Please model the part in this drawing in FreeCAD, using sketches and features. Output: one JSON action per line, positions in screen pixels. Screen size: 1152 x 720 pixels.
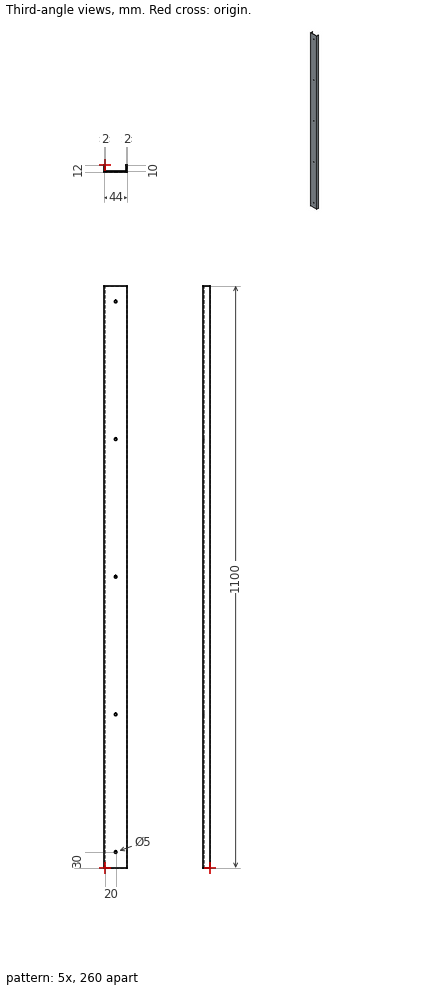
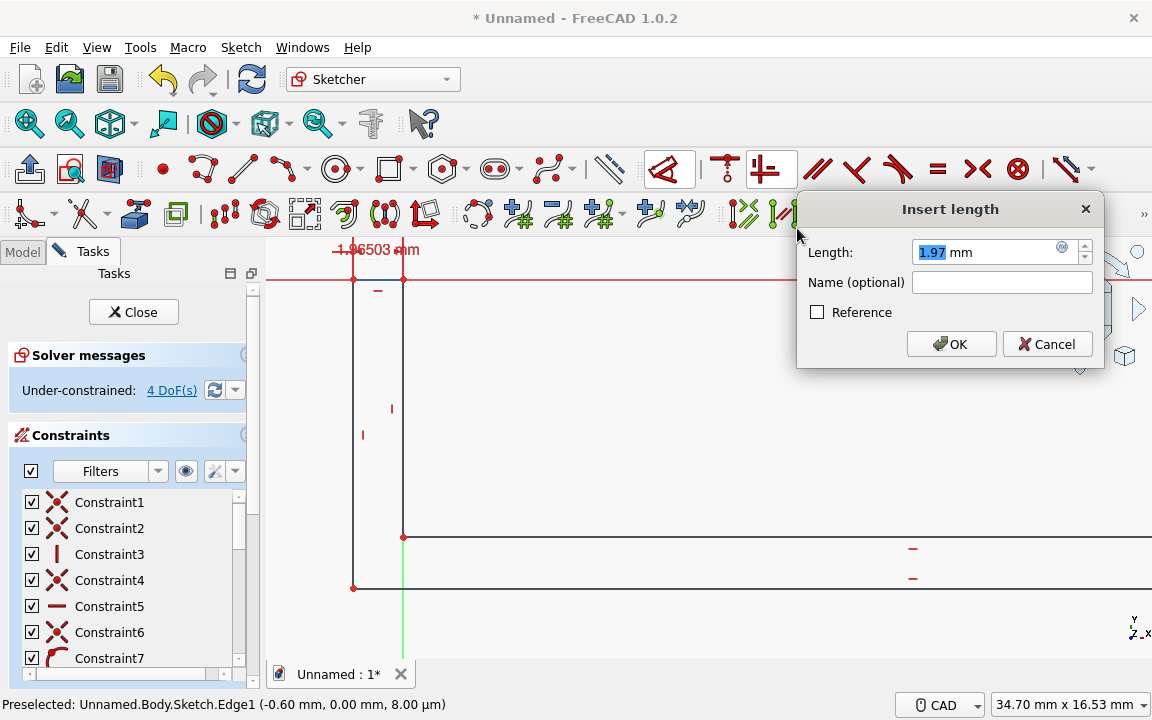
{"action": "type", "text": "2"}
{"action": "key", "text": "Return"}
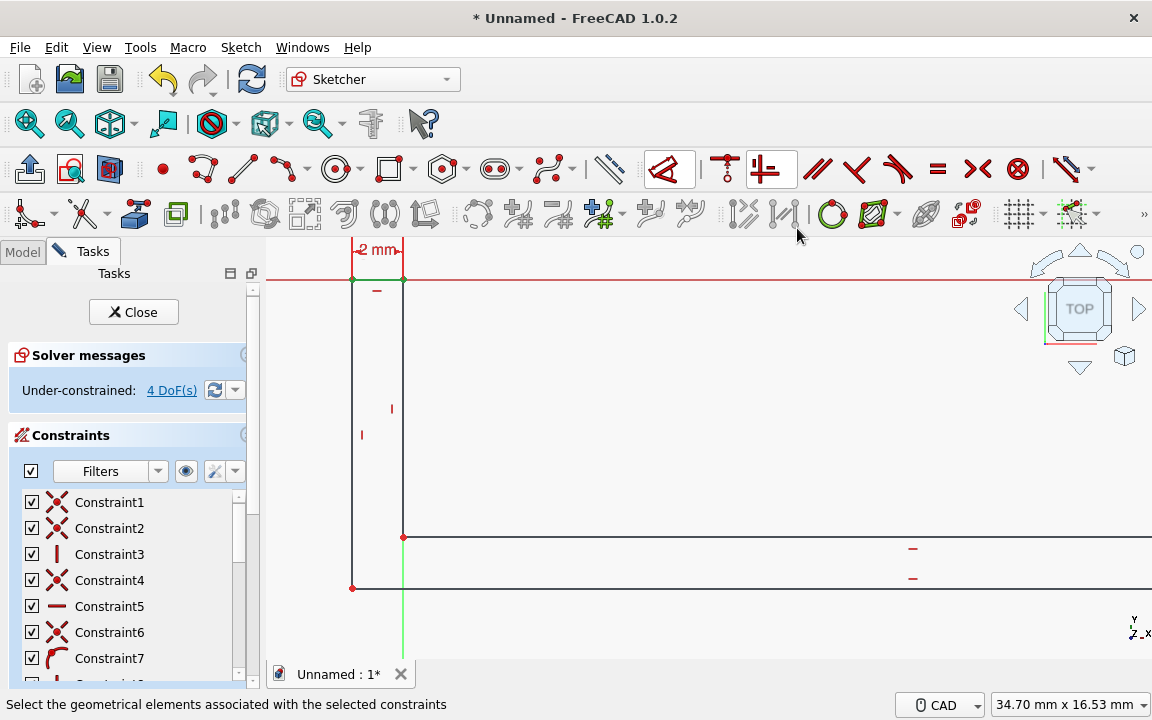
{"action": "scroll", "coordinate": [418, 460], "scroll_direction": "down", "scroll_amount": 4}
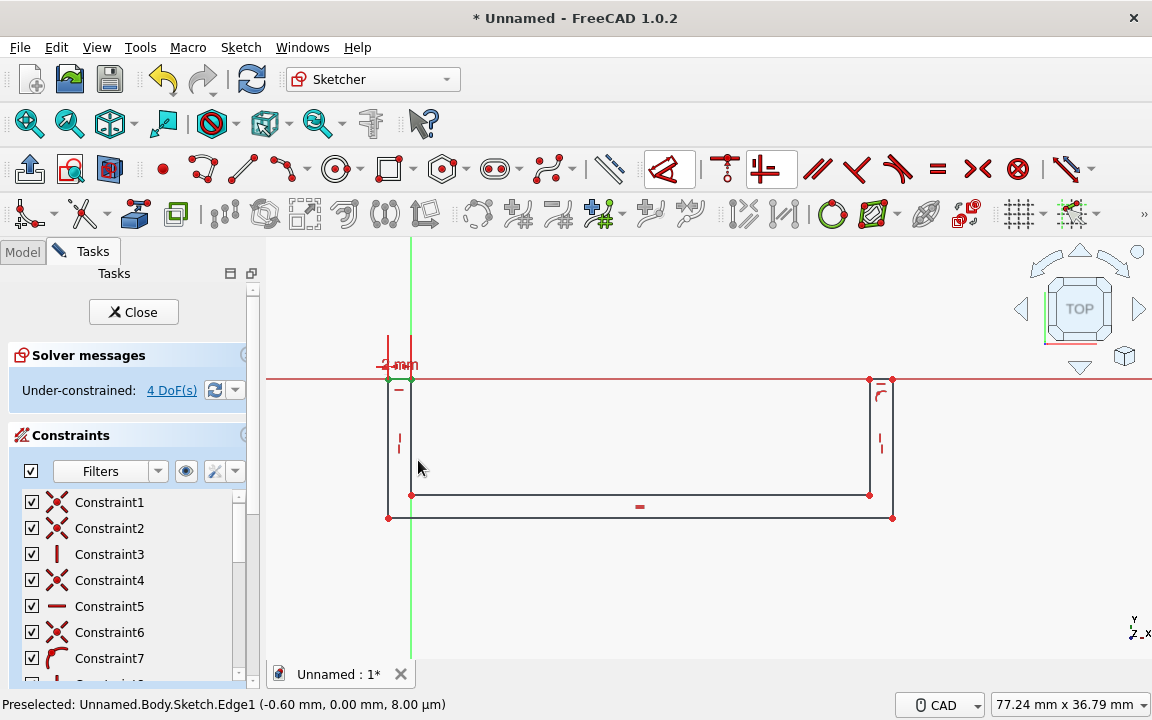
{"action": "scroll", "coordinate": [886, 379], "scroll_direction": "up", "scroll_amount": 4}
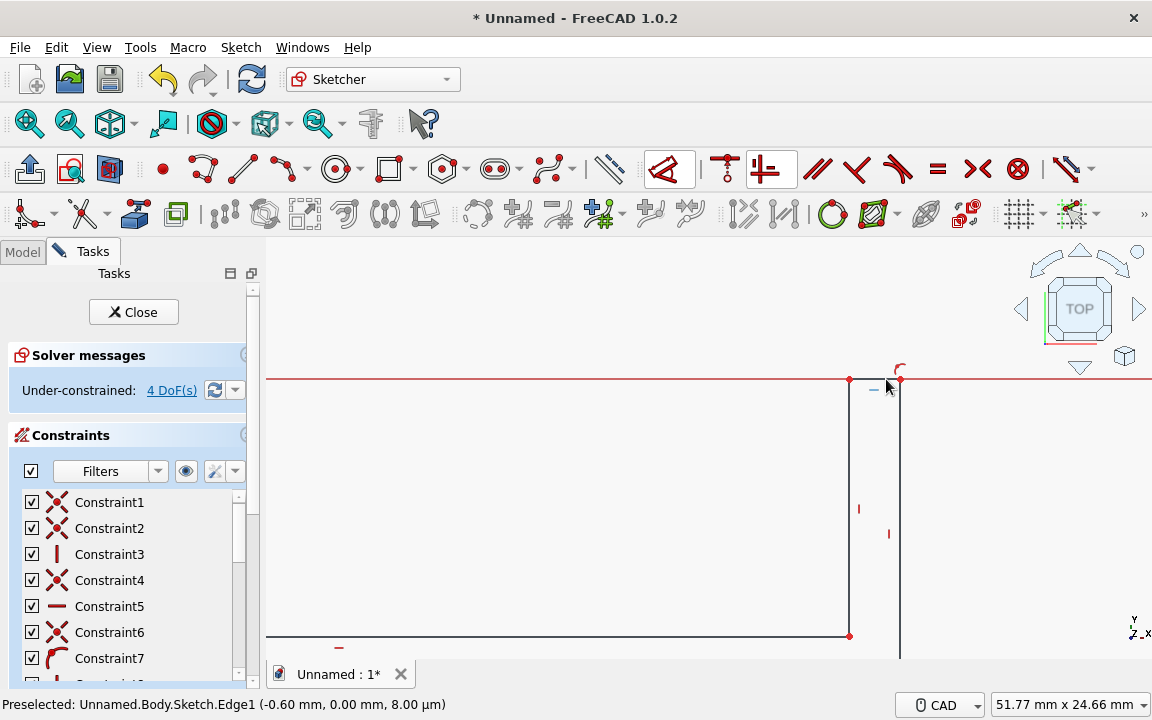
{"action": "left_click", "coordinate": [885, 379]}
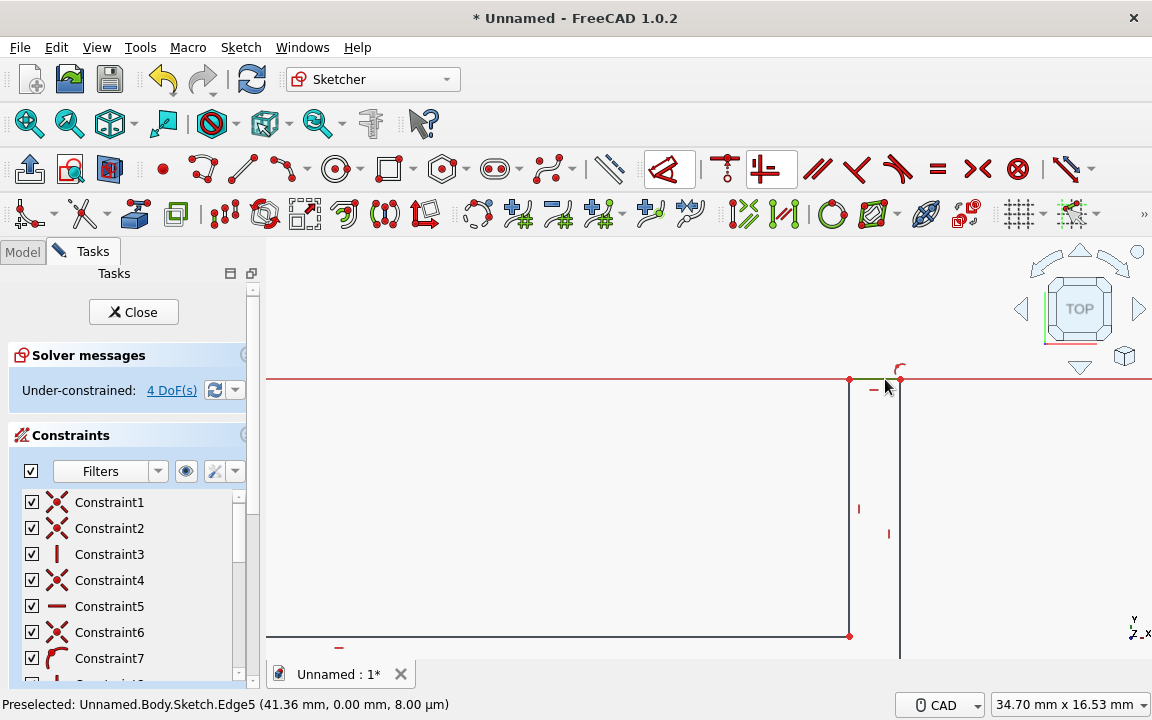
{"action": "key", "text": "l"}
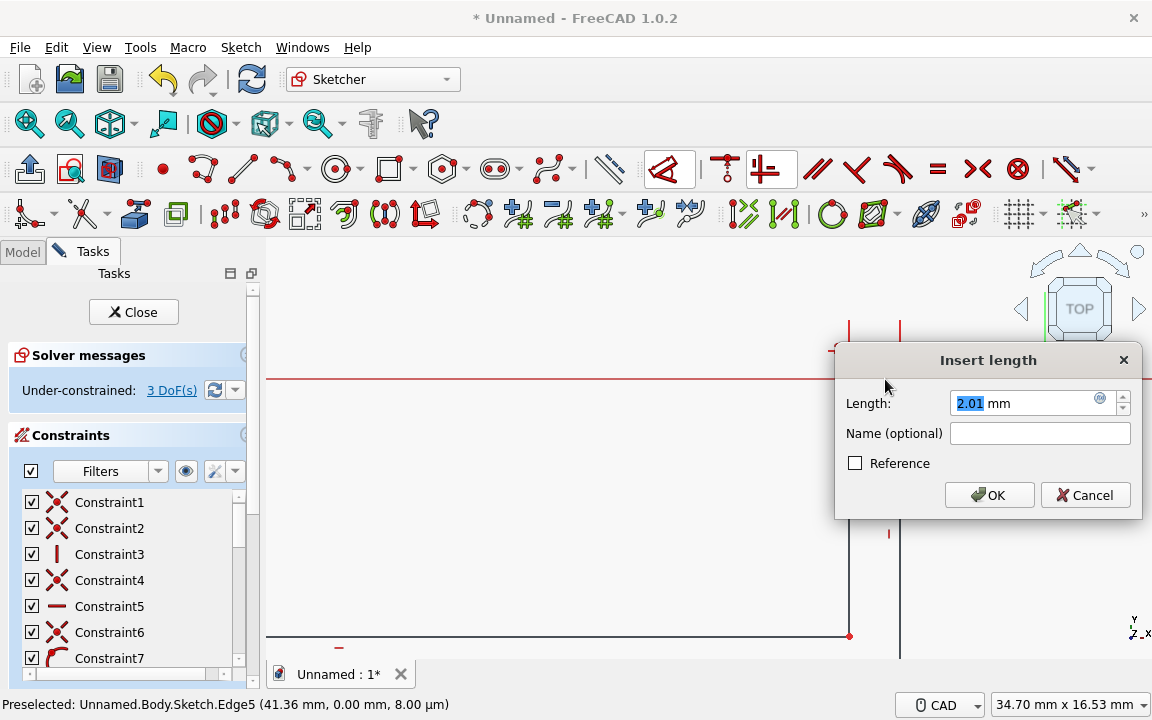
{"action": "type", "text": "2"}
{"action": "key", "text": "Return"}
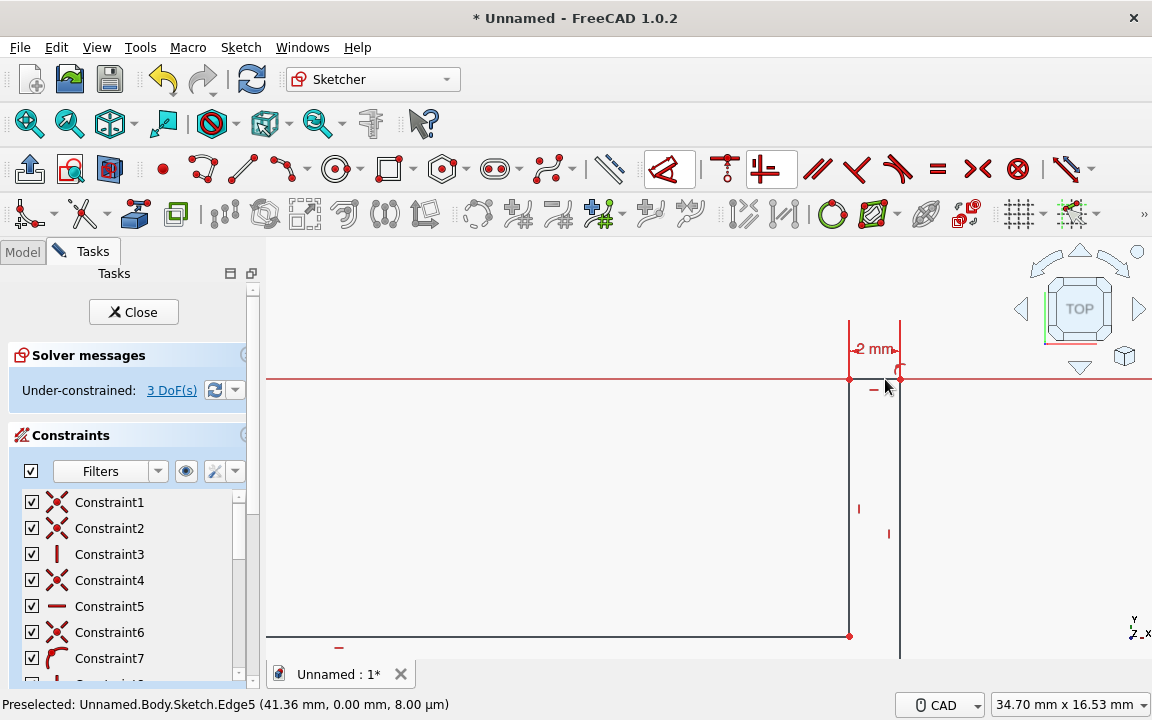
{"action": "scroll", "coordinate": [886, 379], "scroll_direction": "down", "scroll_amount": 4}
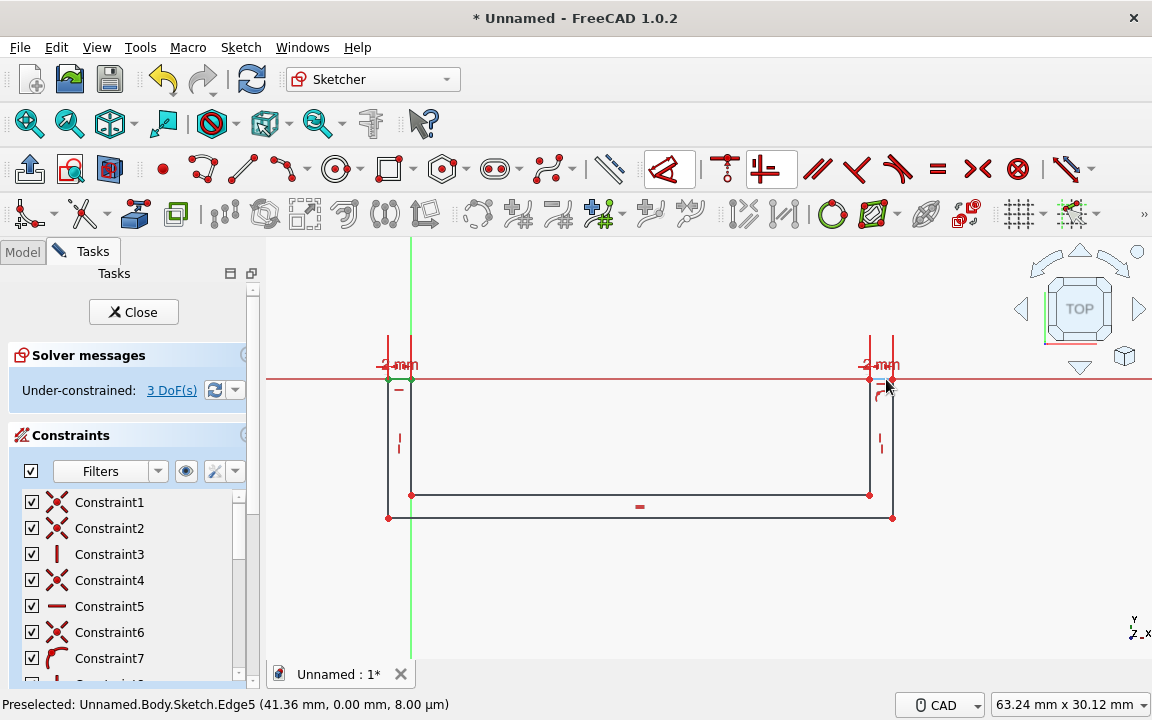
{"action": "left_click", "coordinate": [388, 421]}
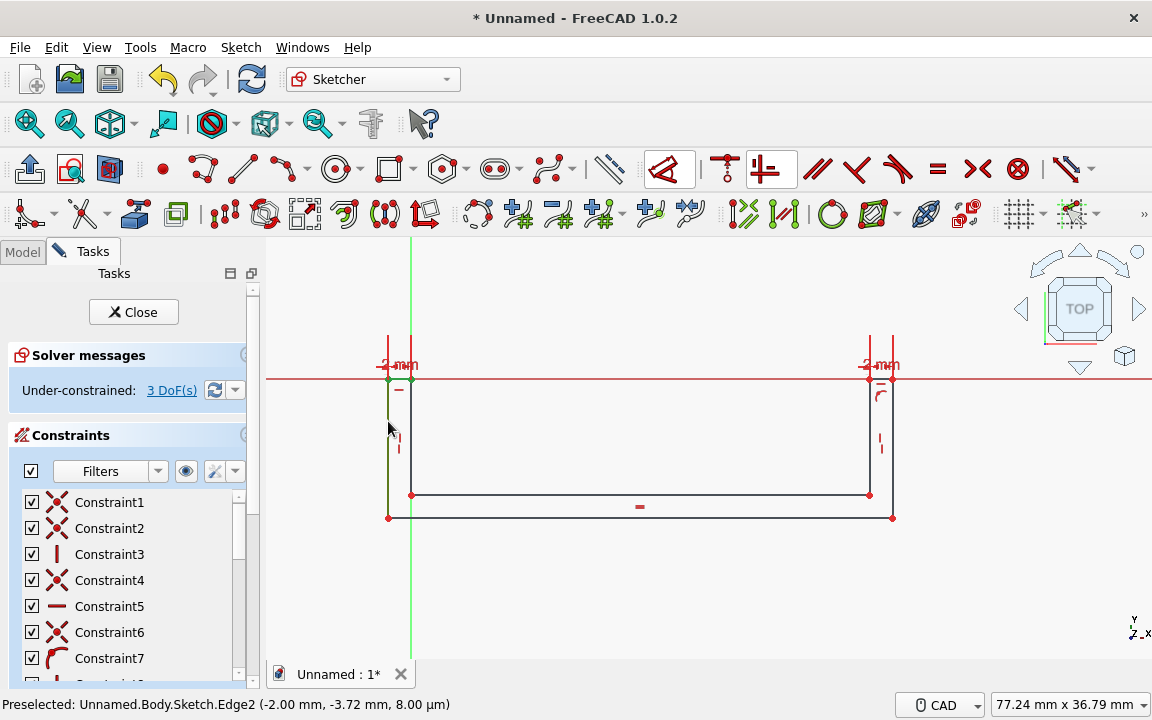
{"action": "left_click", "coordinate": [690, 170]}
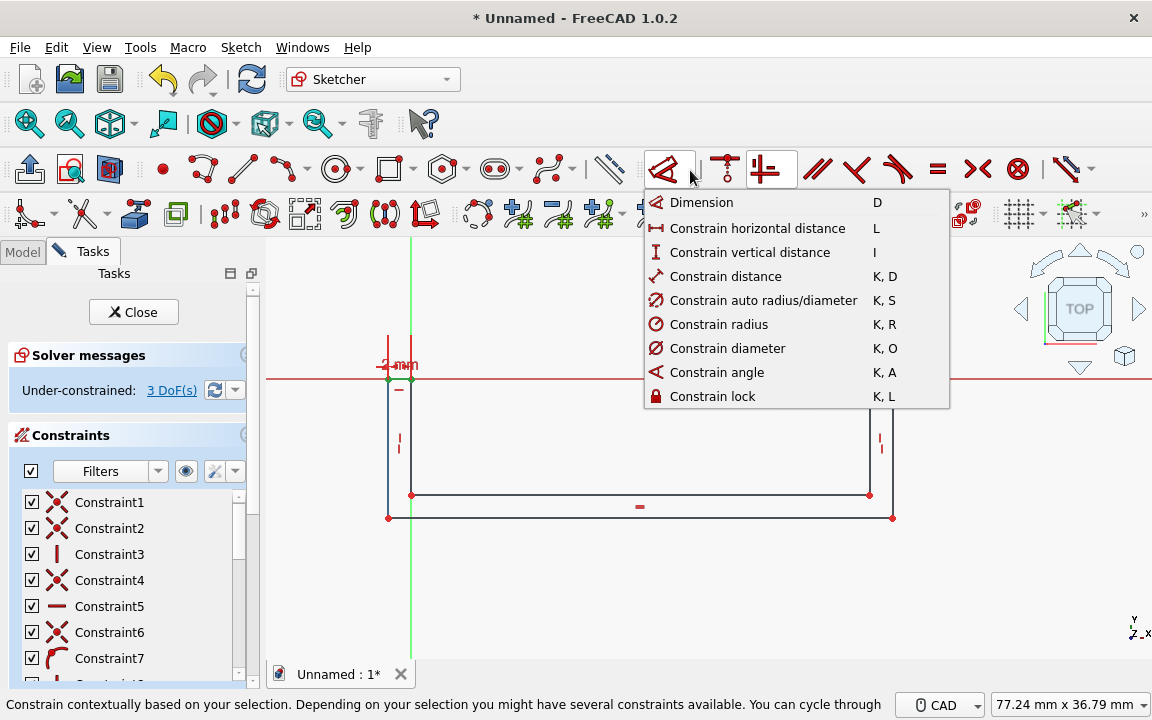
{"action": "left_click", "coordinate": [797, 252]}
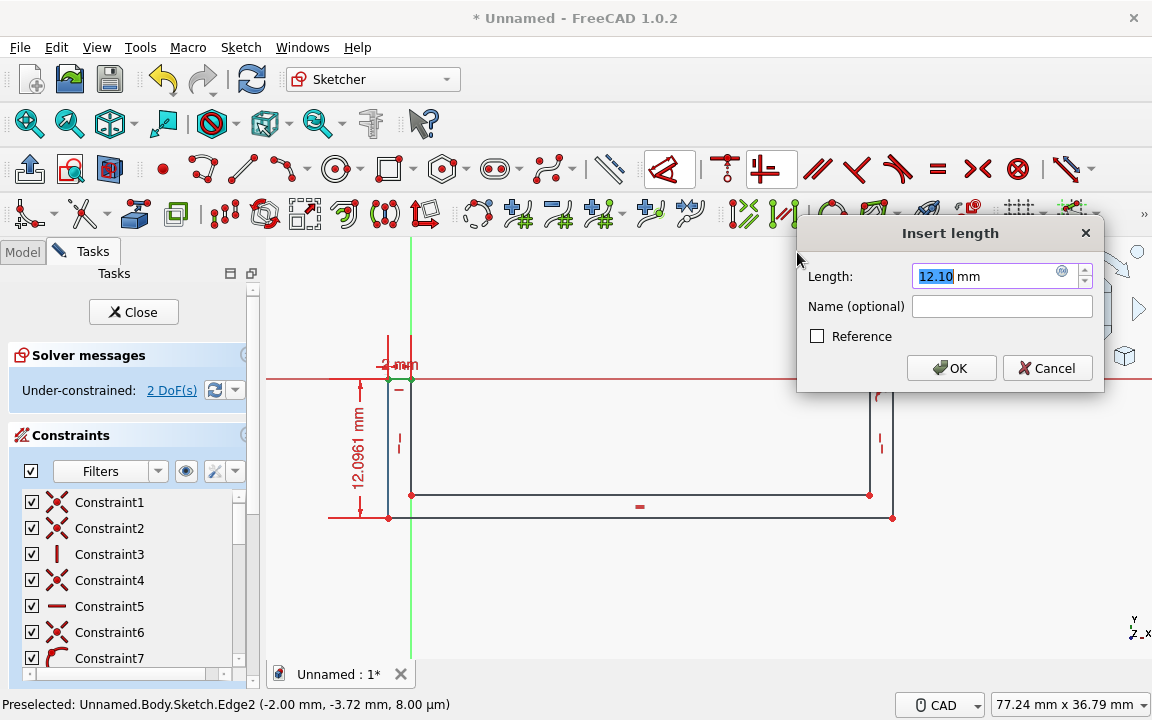
{"action": "type", "text": "12"}
{"action": "key", "text": "Return"}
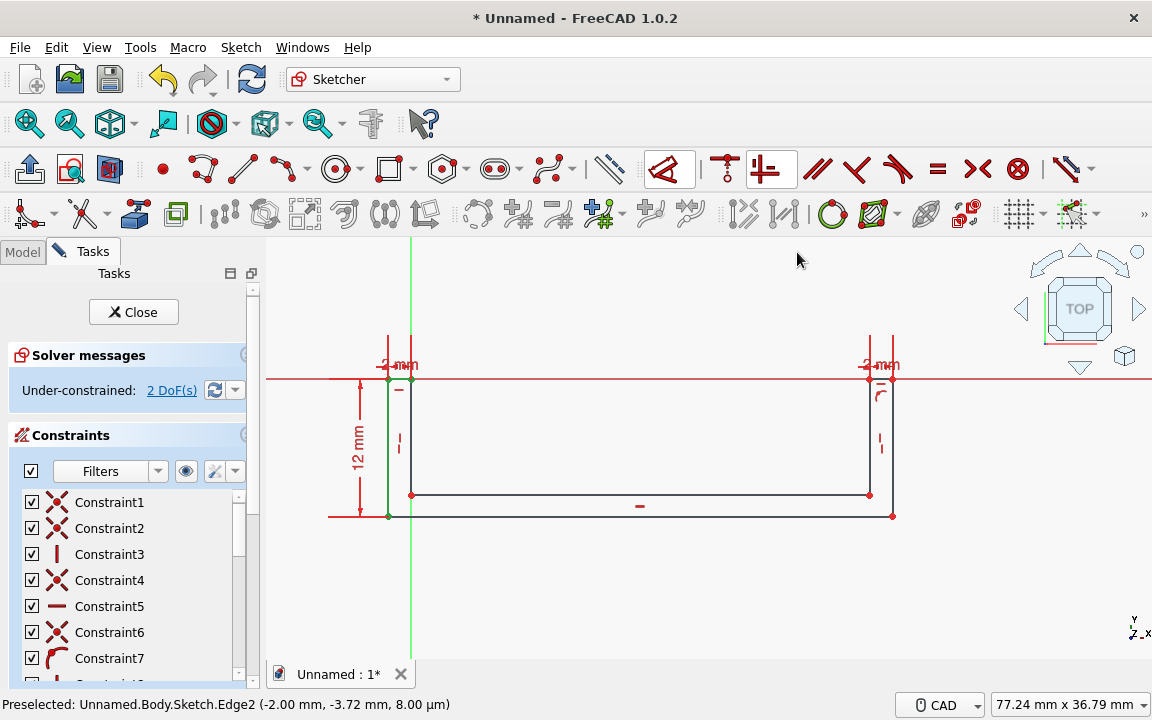
{"action": "left_click", "coordinate": [540, 517]}